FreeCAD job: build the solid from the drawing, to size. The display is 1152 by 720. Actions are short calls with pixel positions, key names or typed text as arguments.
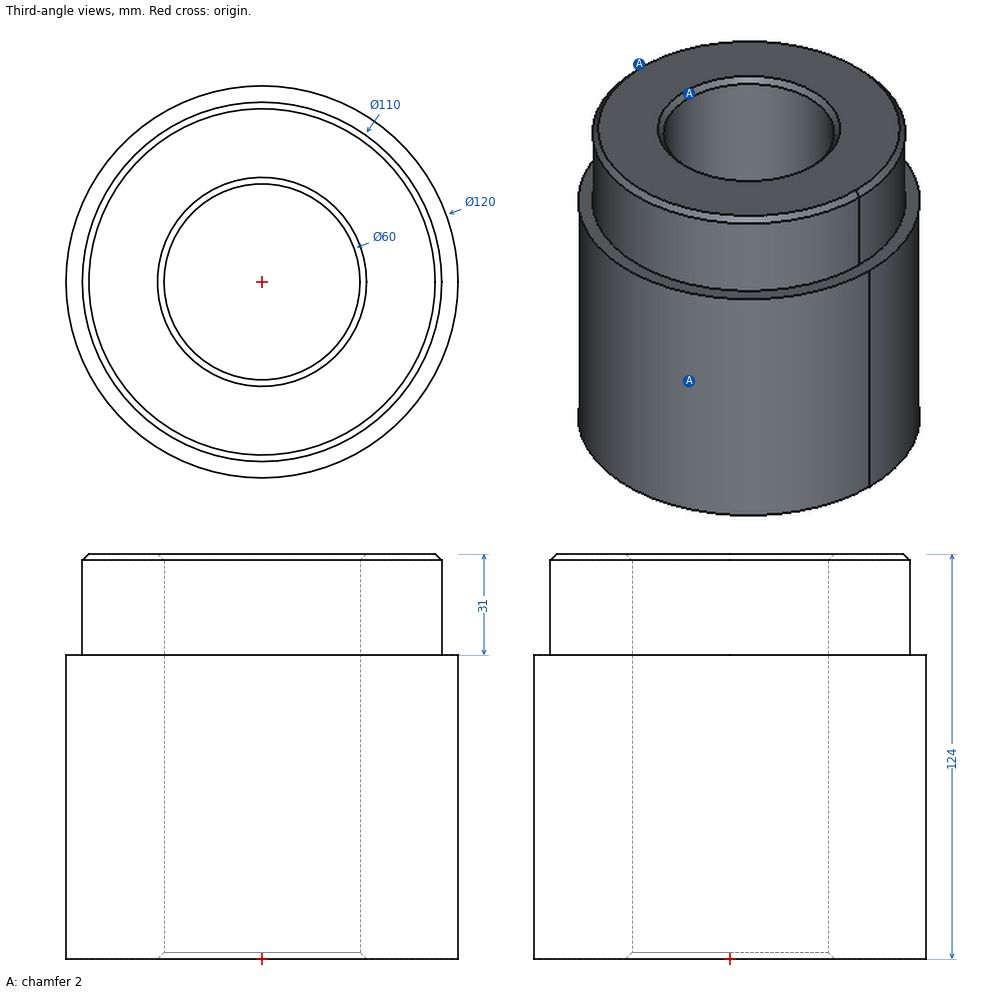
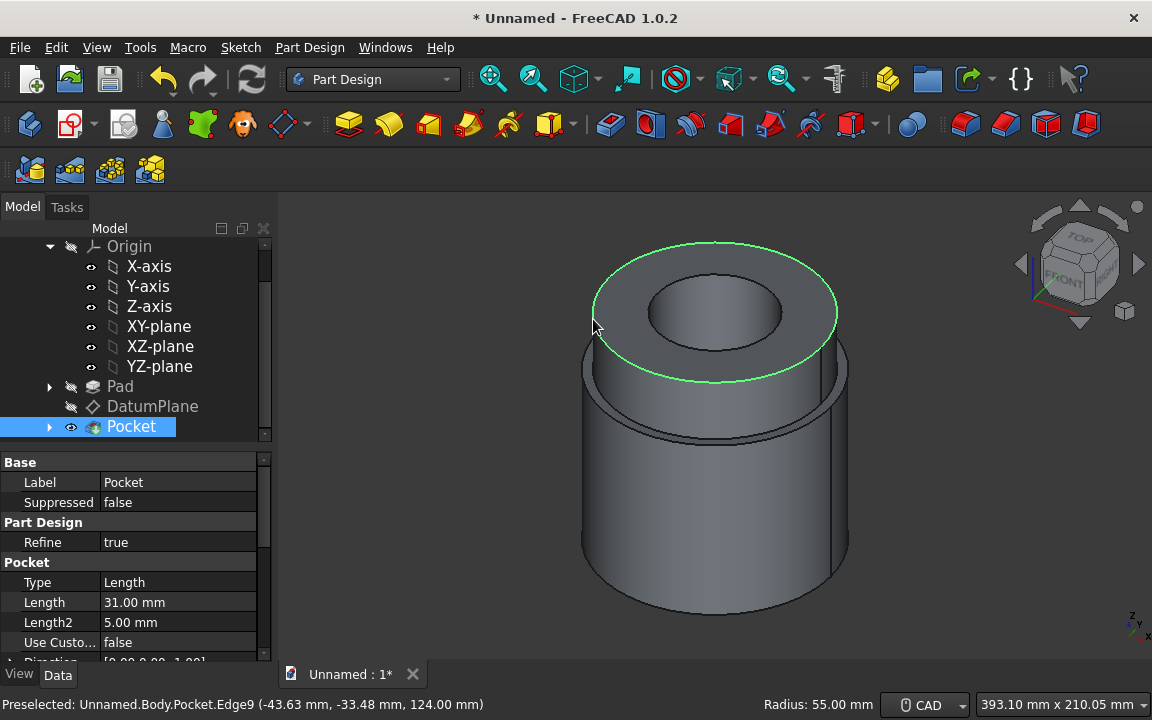
click(657, 292, ctrl)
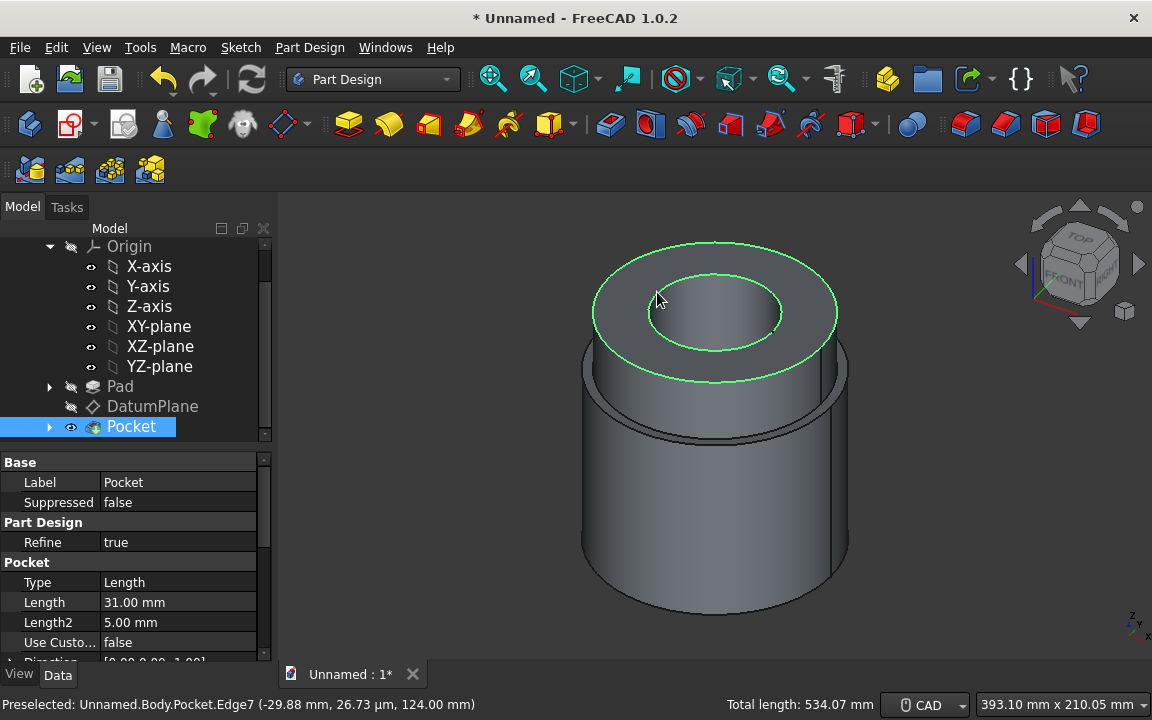
key(0)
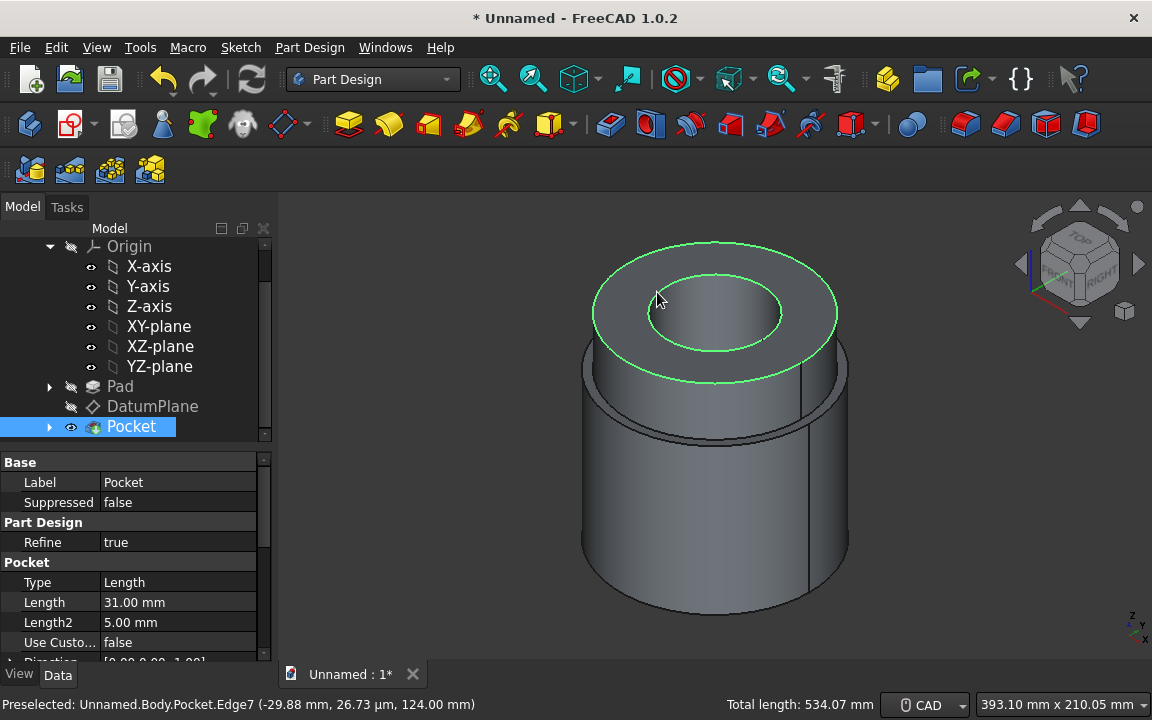
key(2)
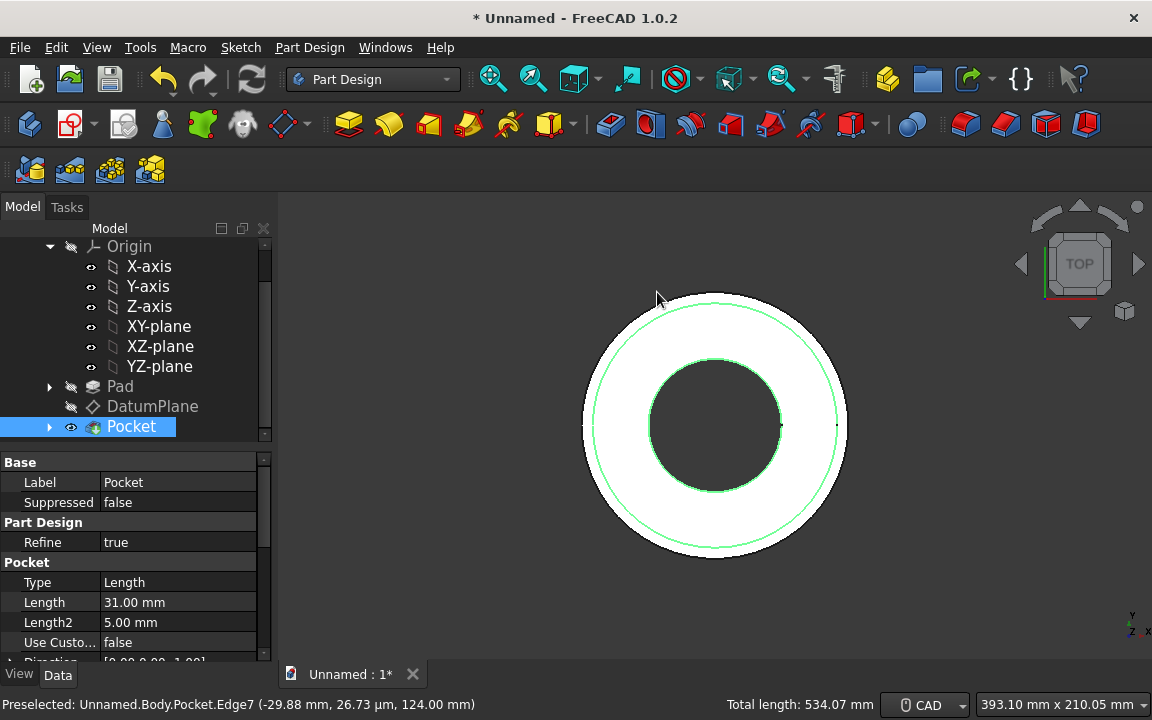
key(1)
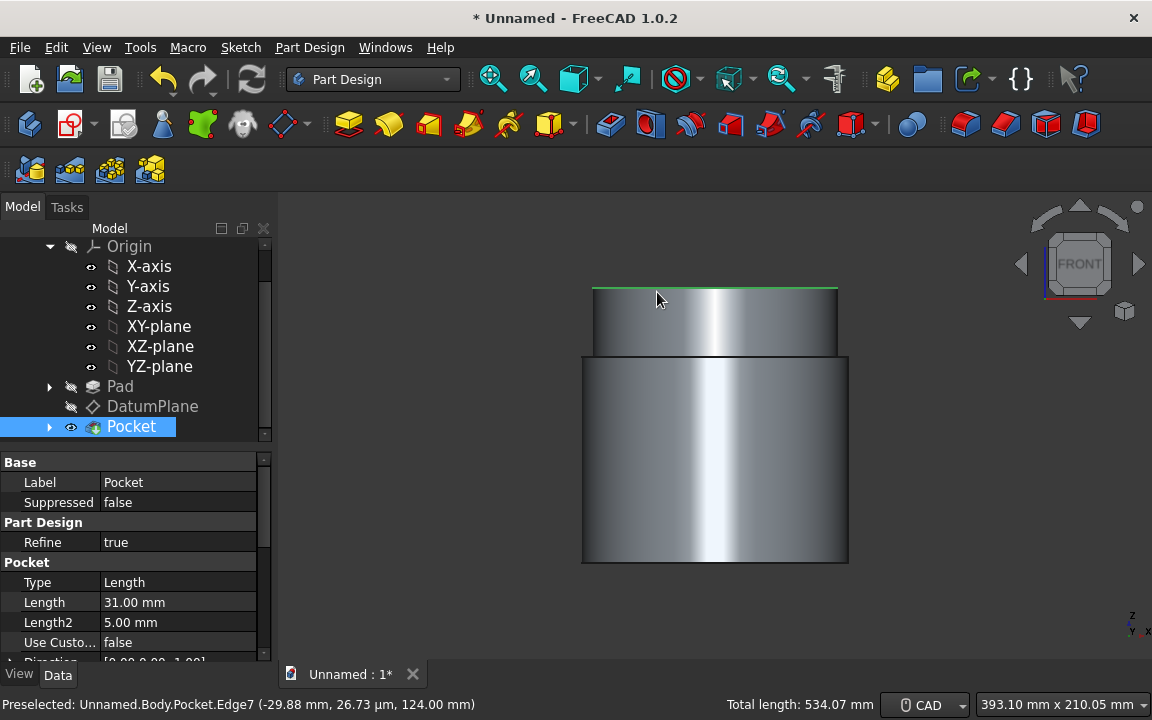
key(3)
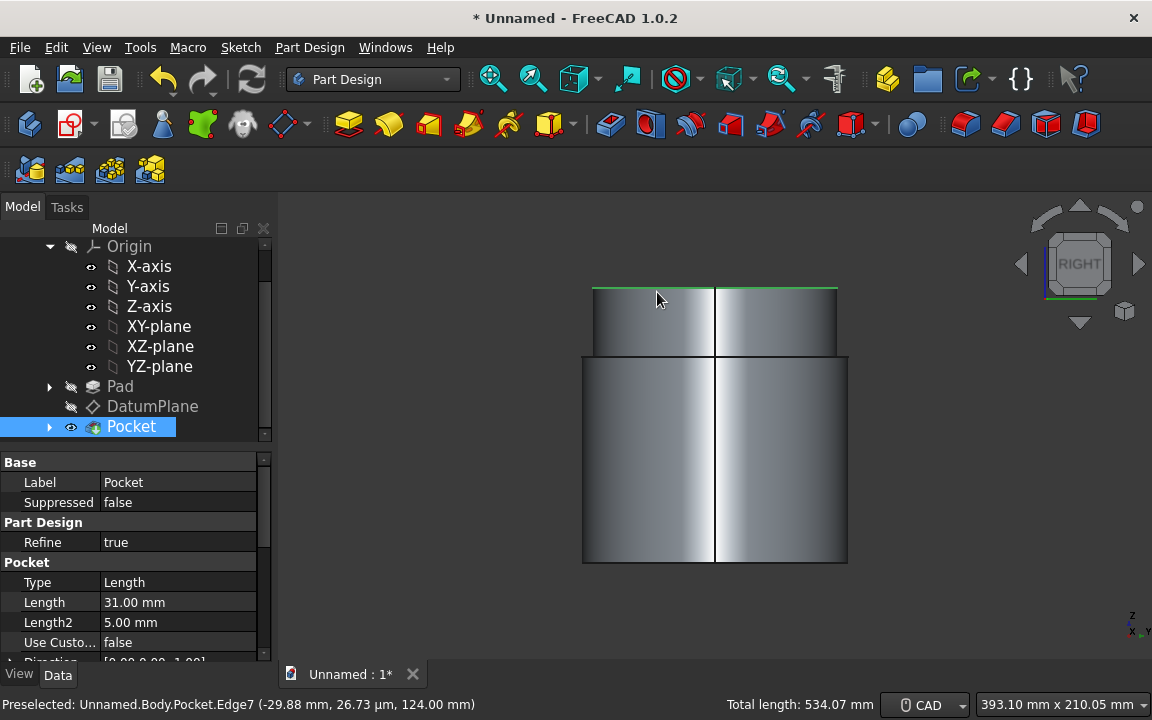
key(5)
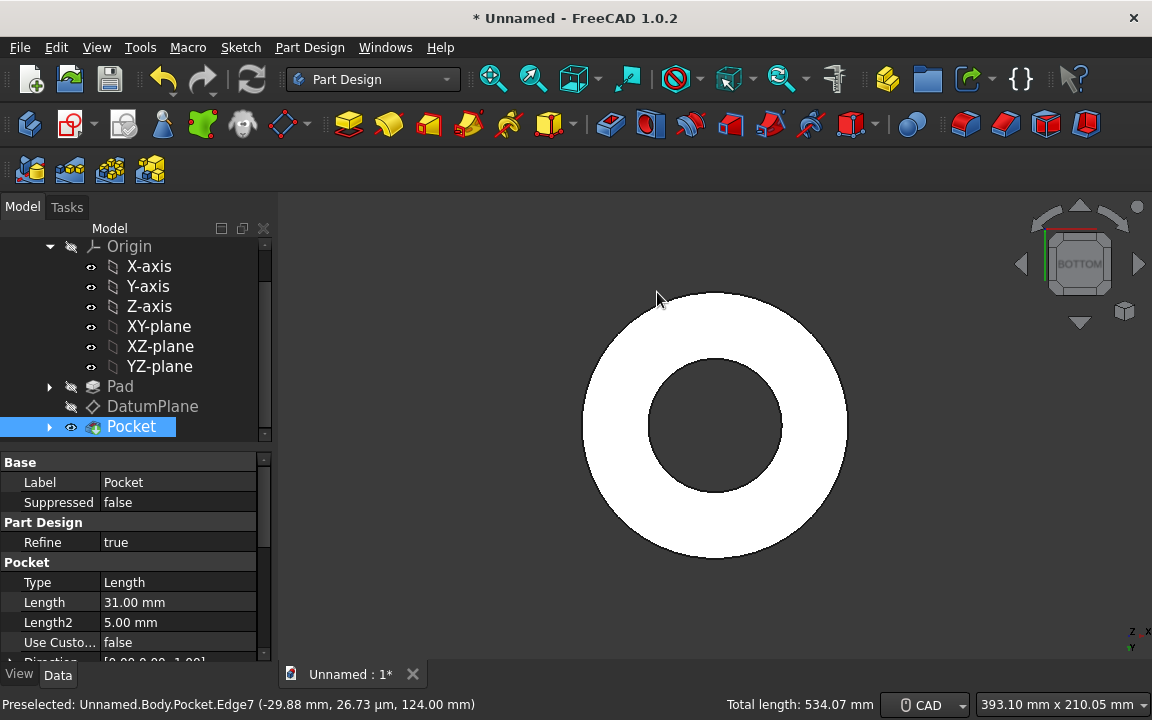
click(648, 424, ctrl)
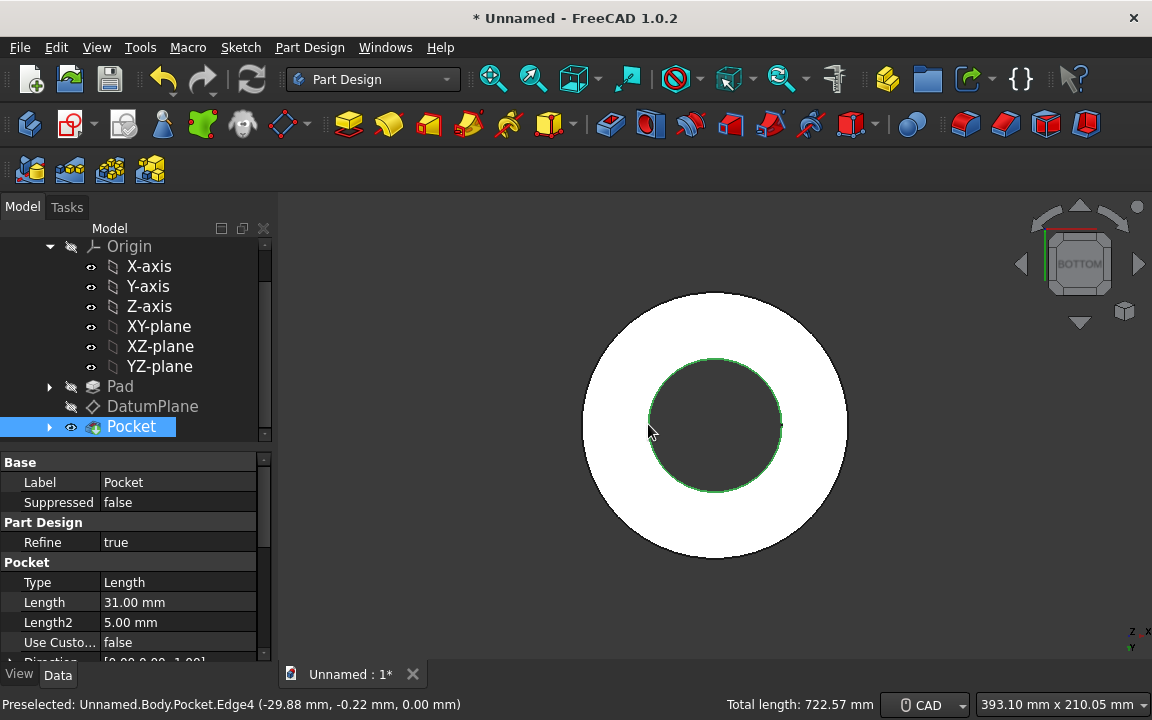
click(1006, 124)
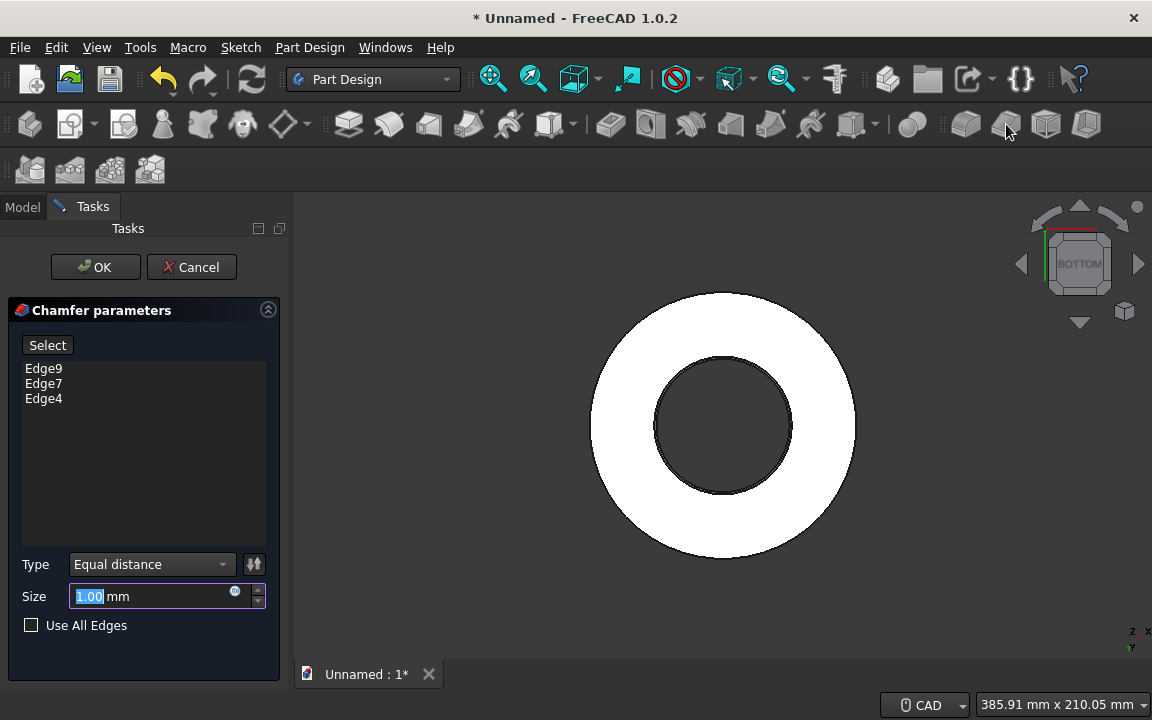
text(2)
key(Tab)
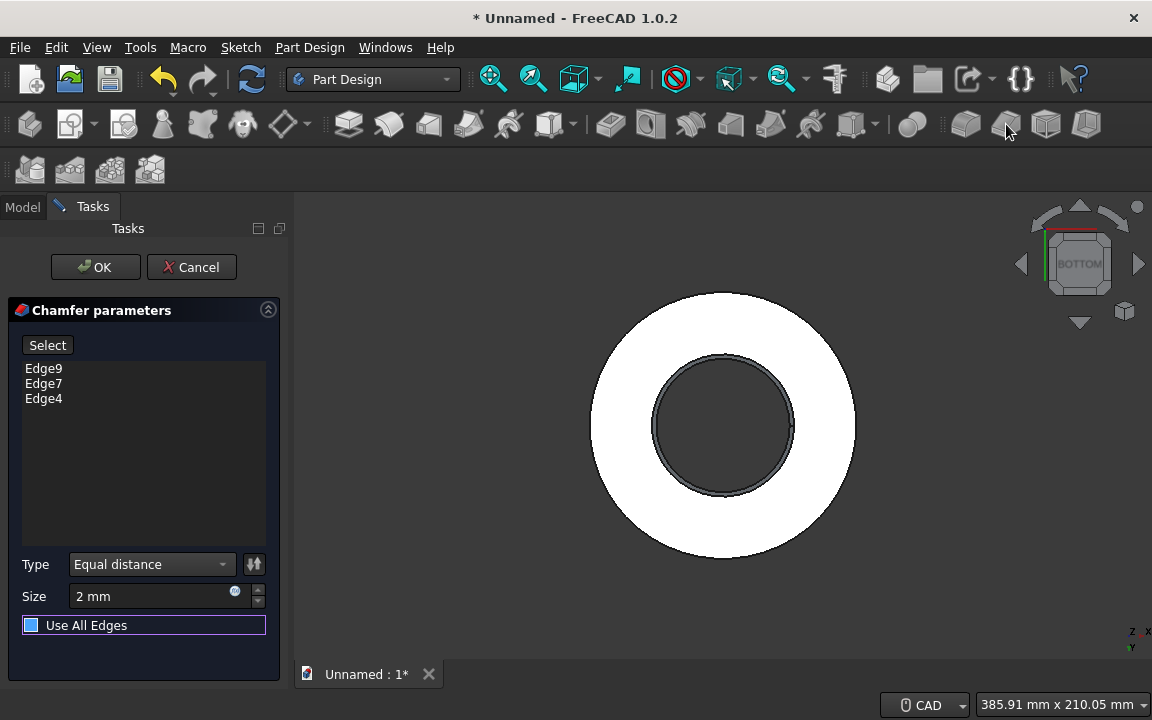
click(96, 267)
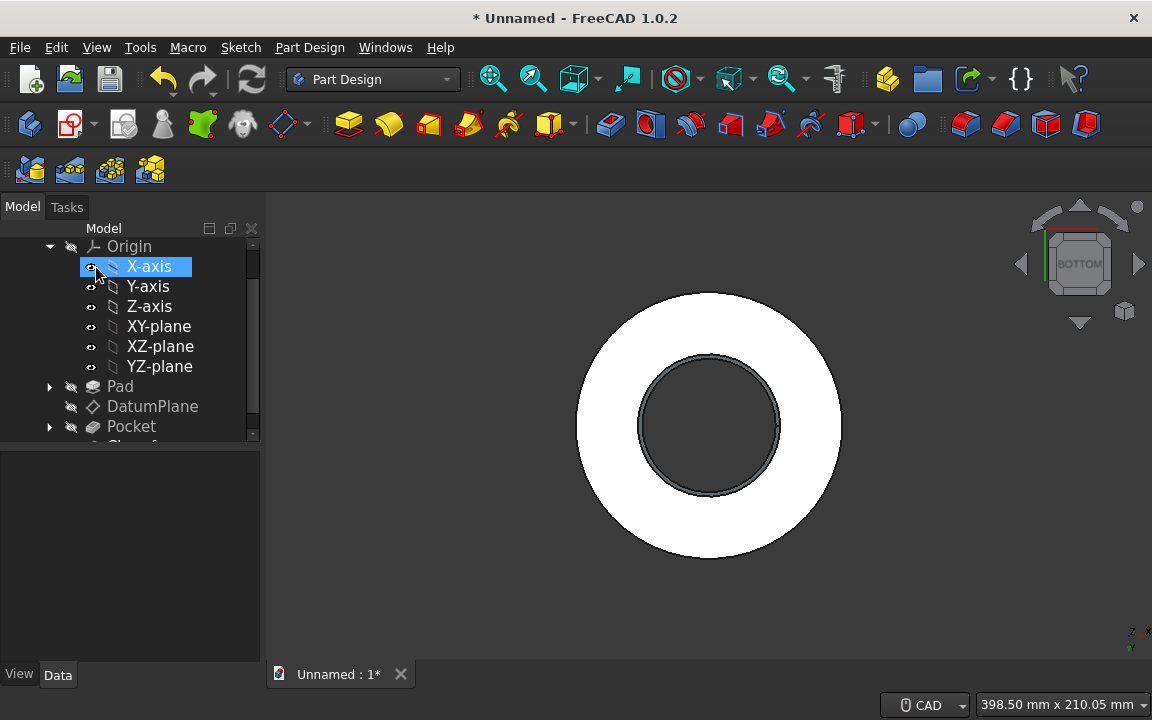
key(0)